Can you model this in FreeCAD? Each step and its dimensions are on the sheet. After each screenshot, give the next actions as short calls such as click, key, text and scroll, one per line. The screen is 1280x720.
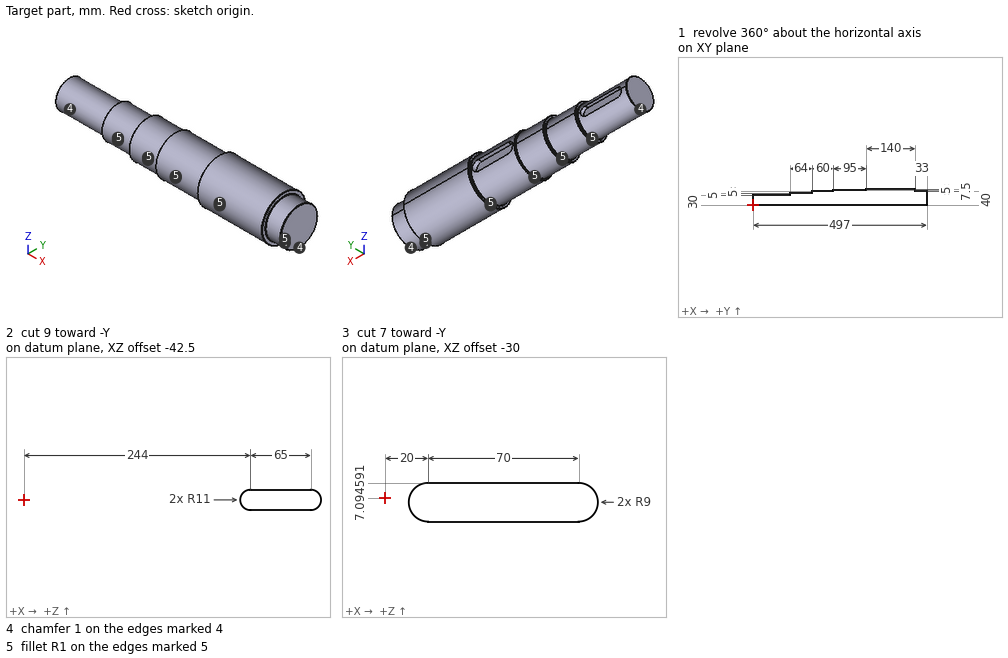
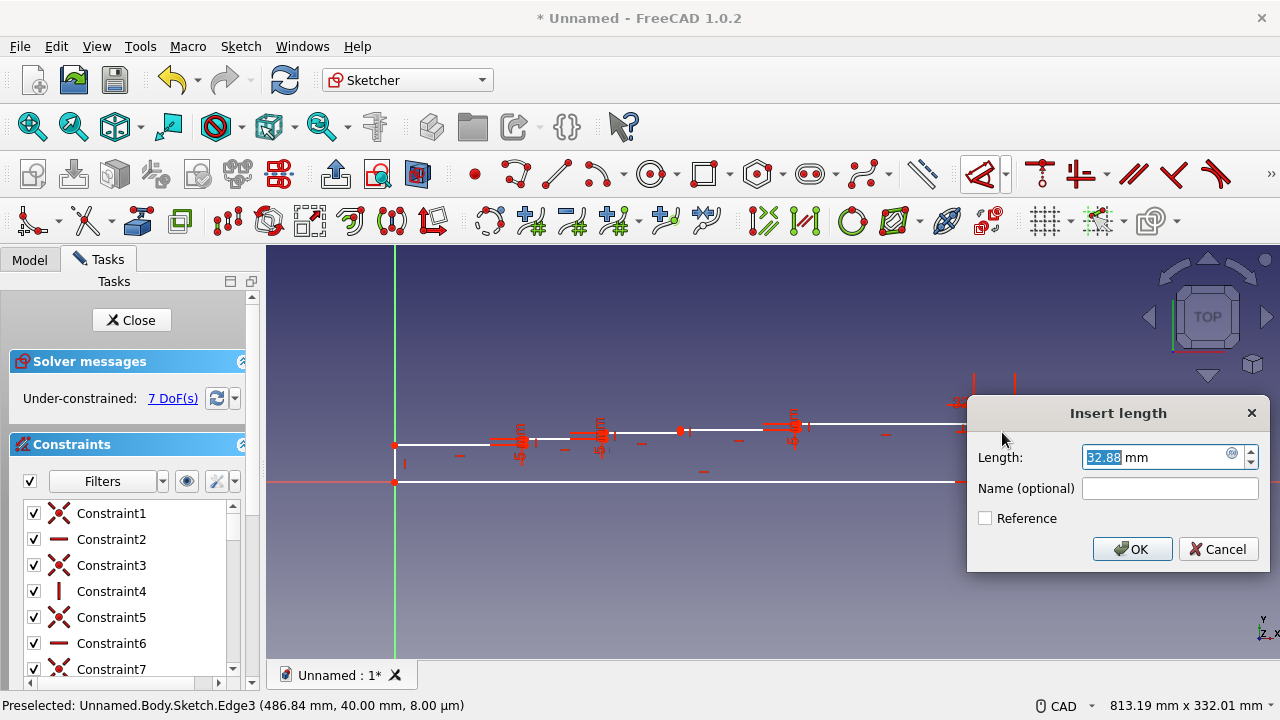
text(33)
key(Return)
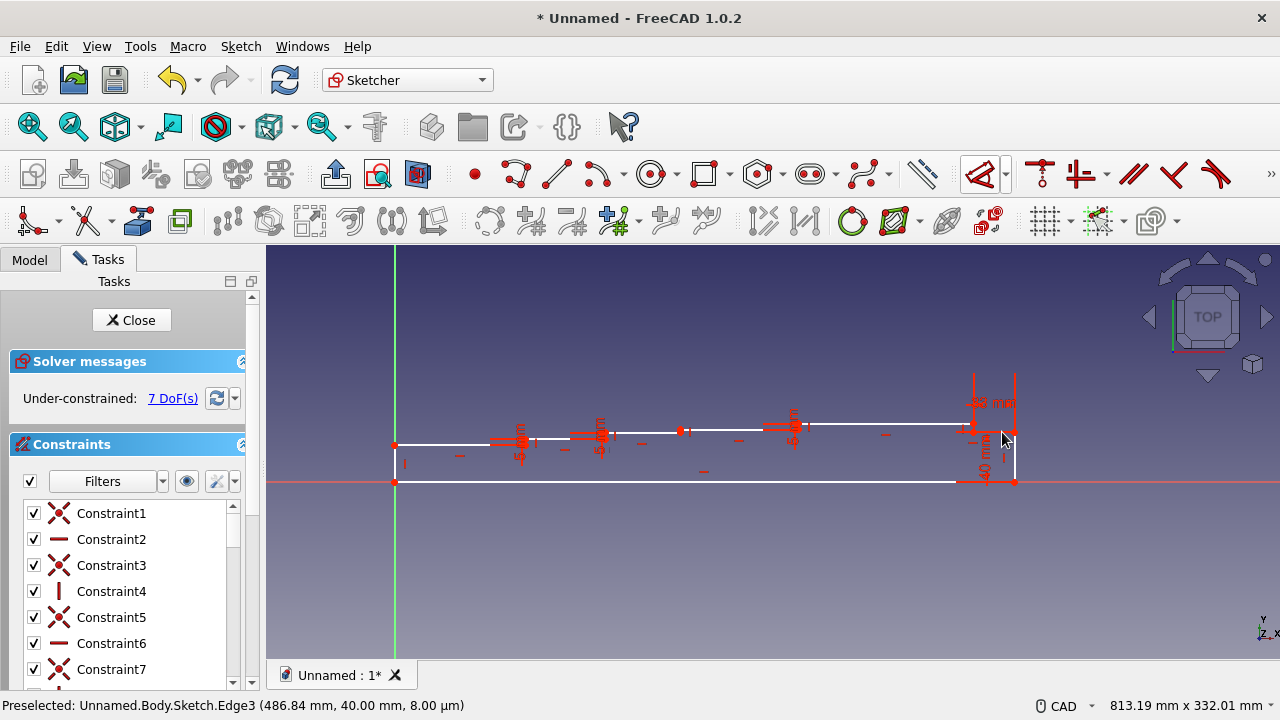
click(763, 430)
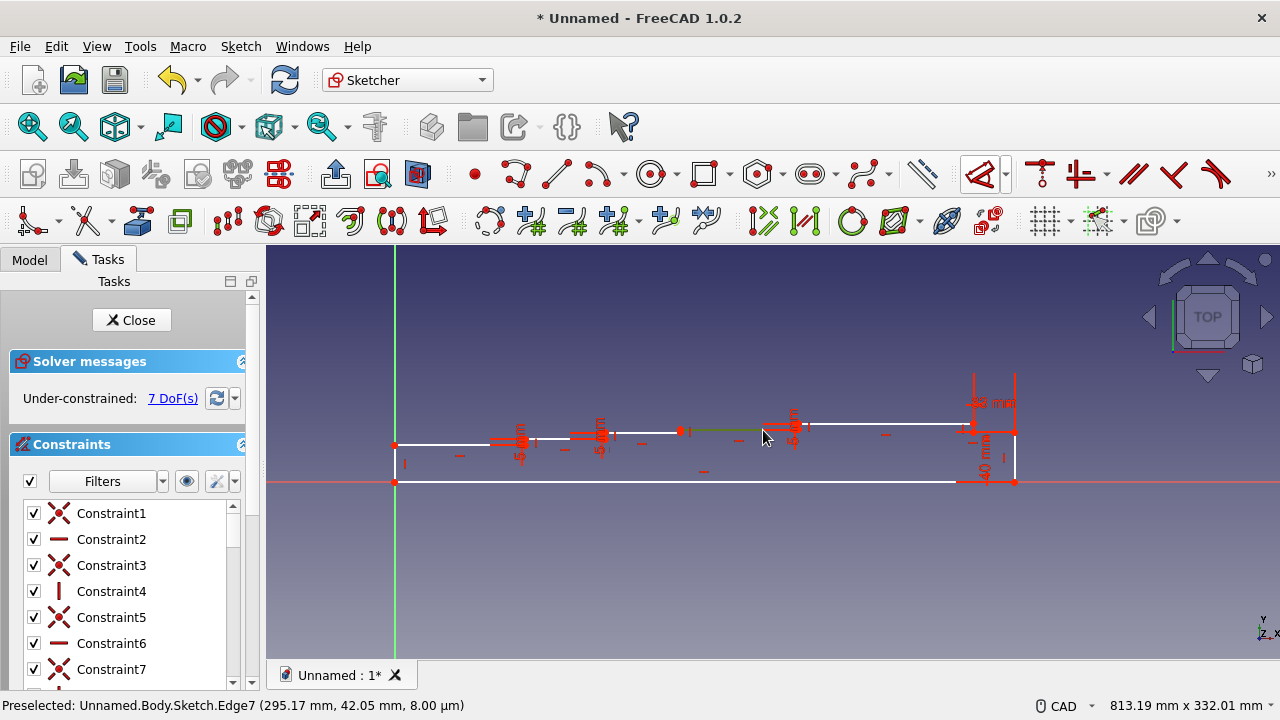
click(1006, 174)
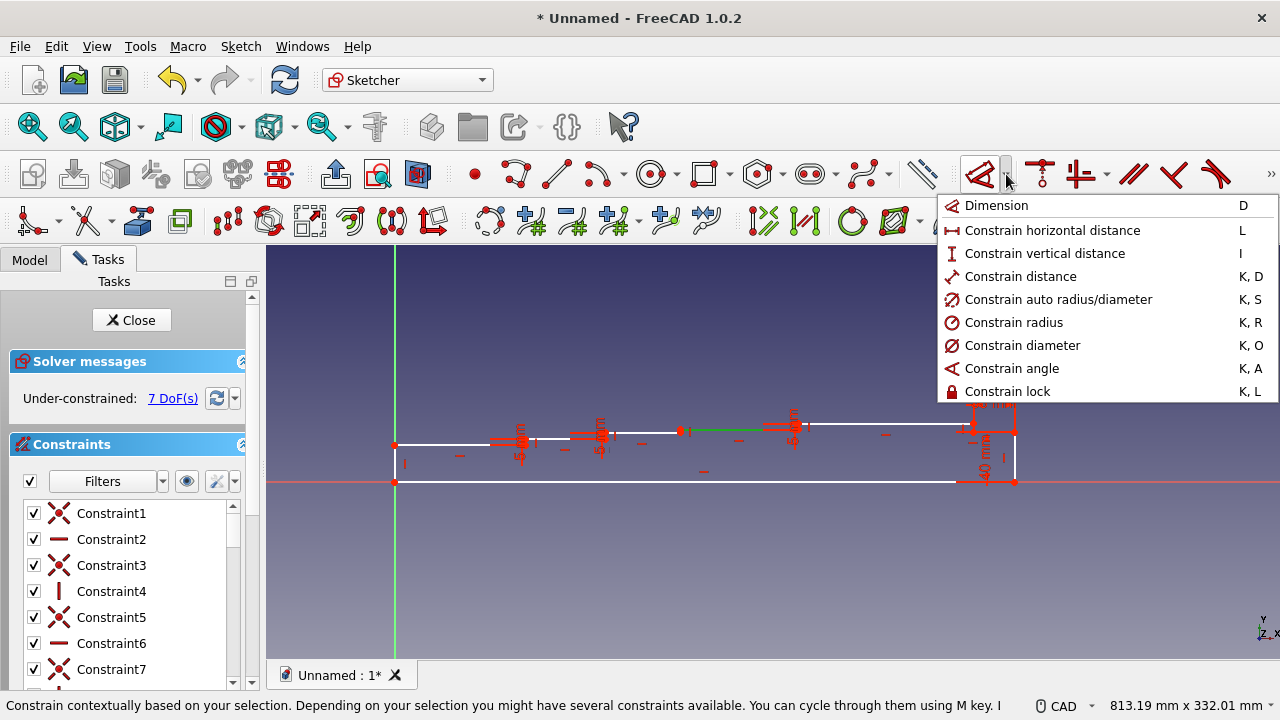
click(1108, 230)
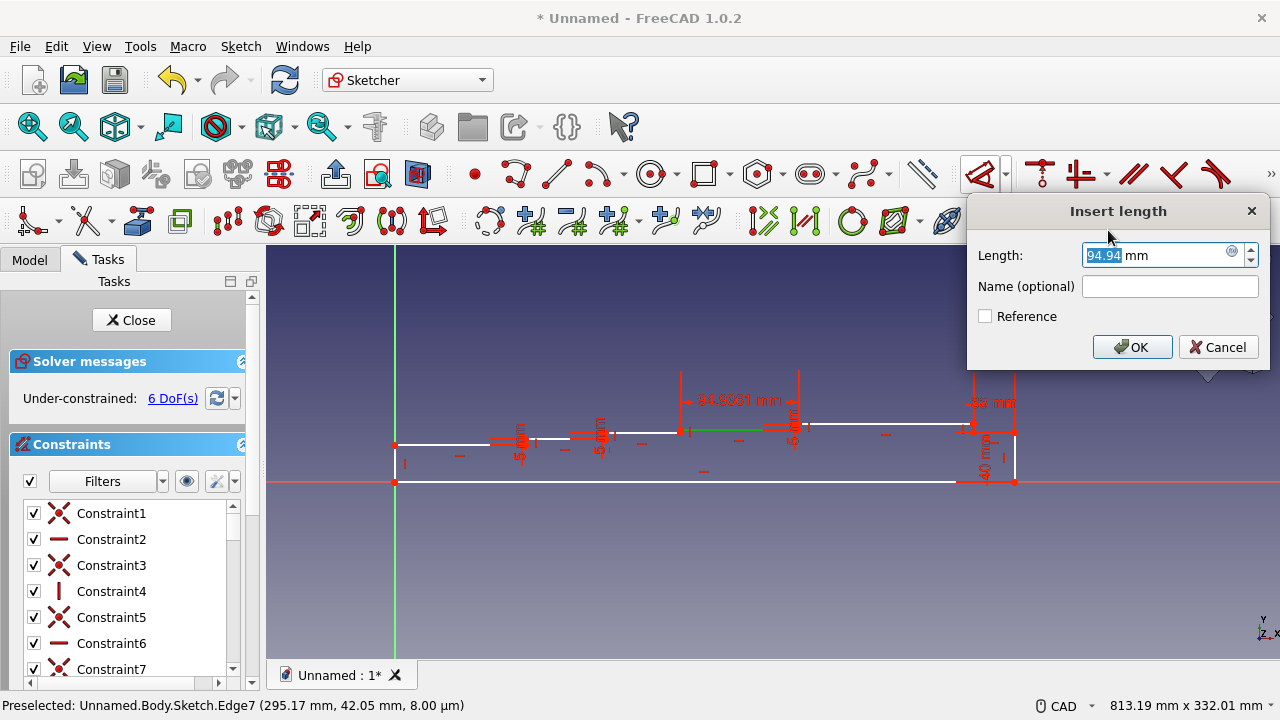
text(95)
key(Return)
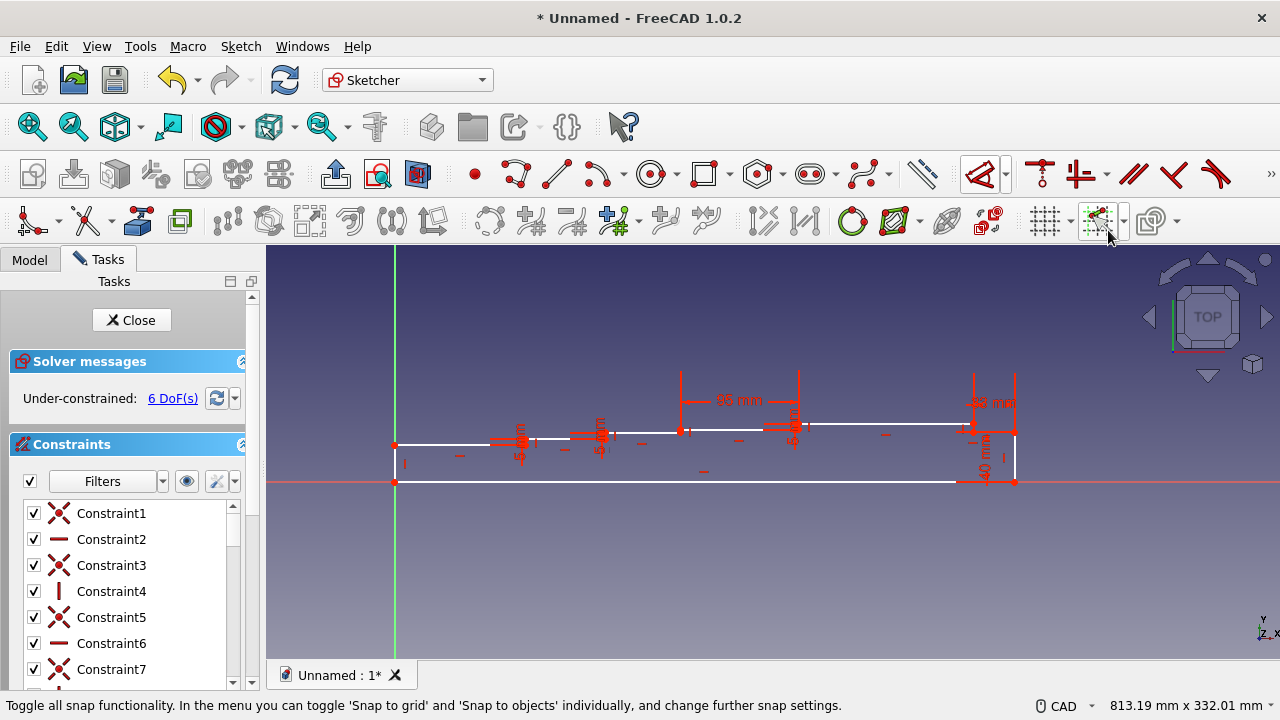
click(658, 433)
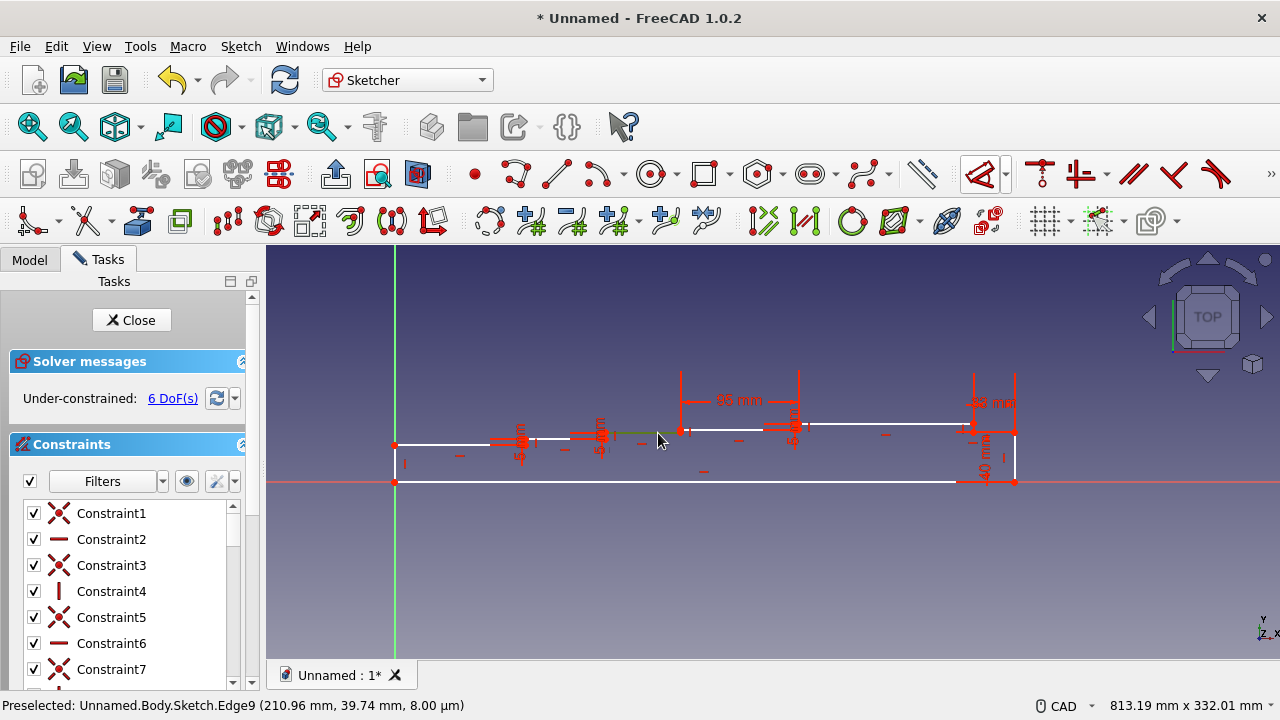
key(l)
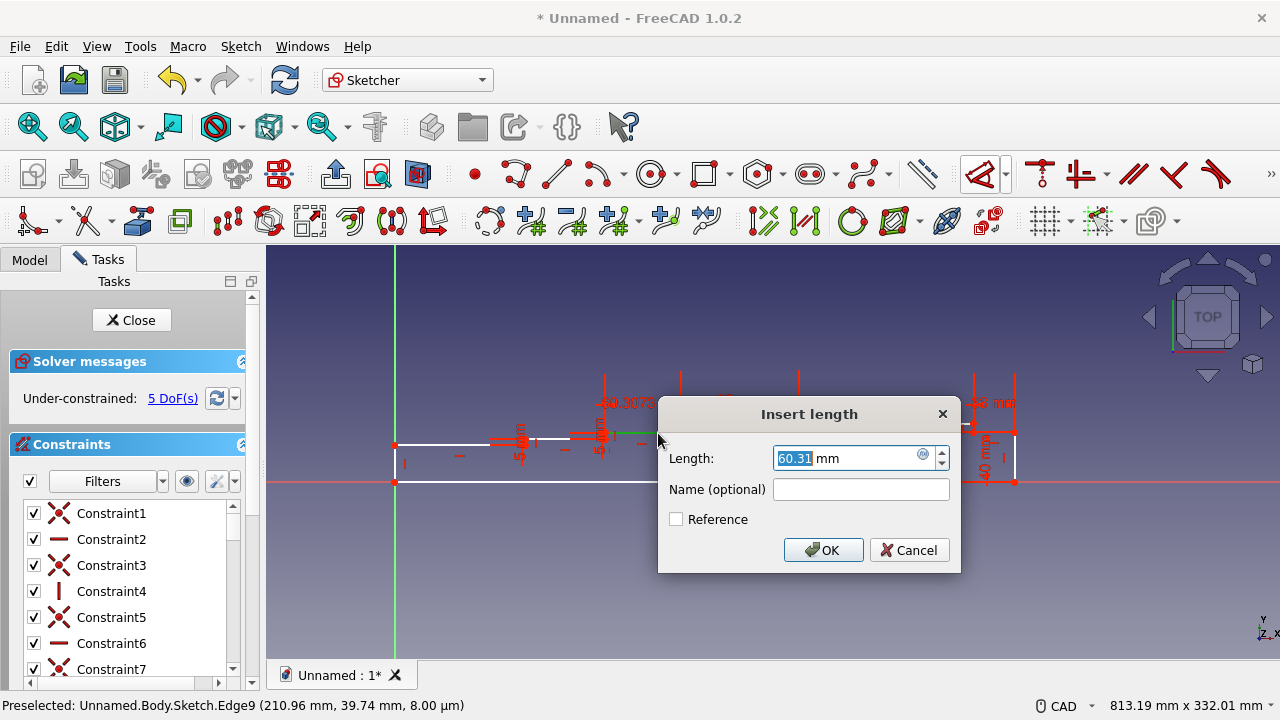
text(60)
key(Return)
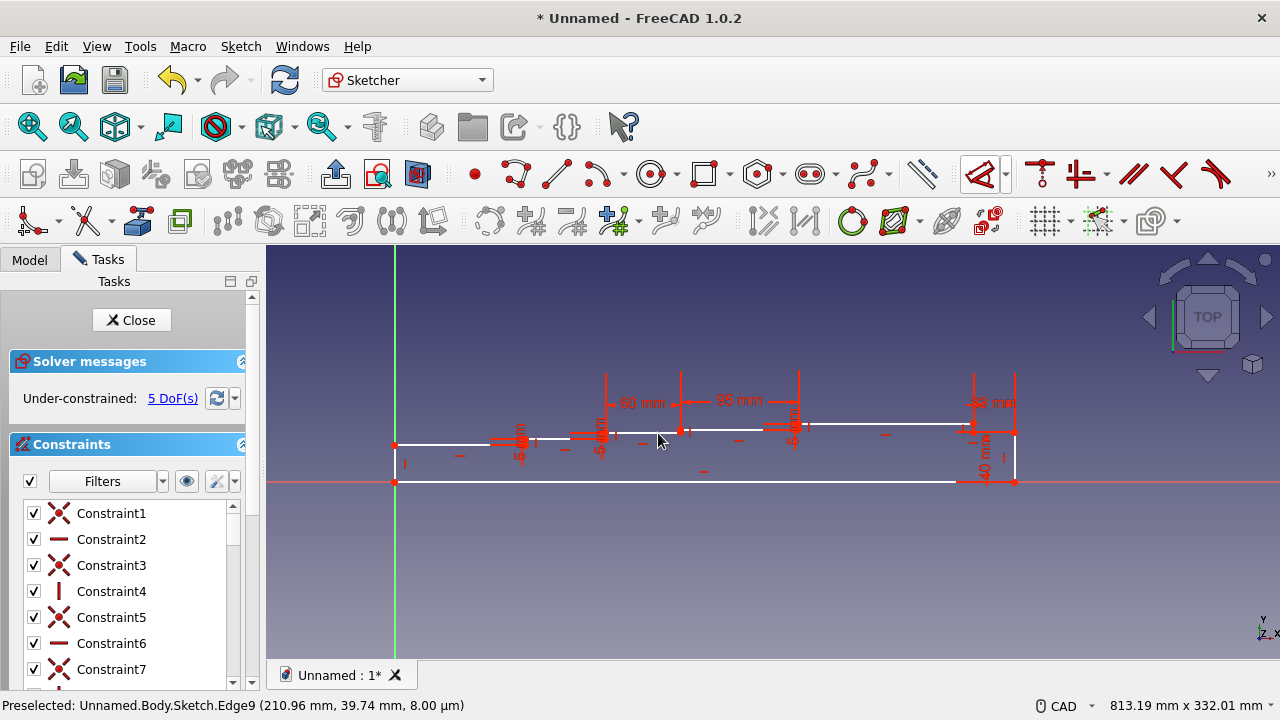
click(582, 439)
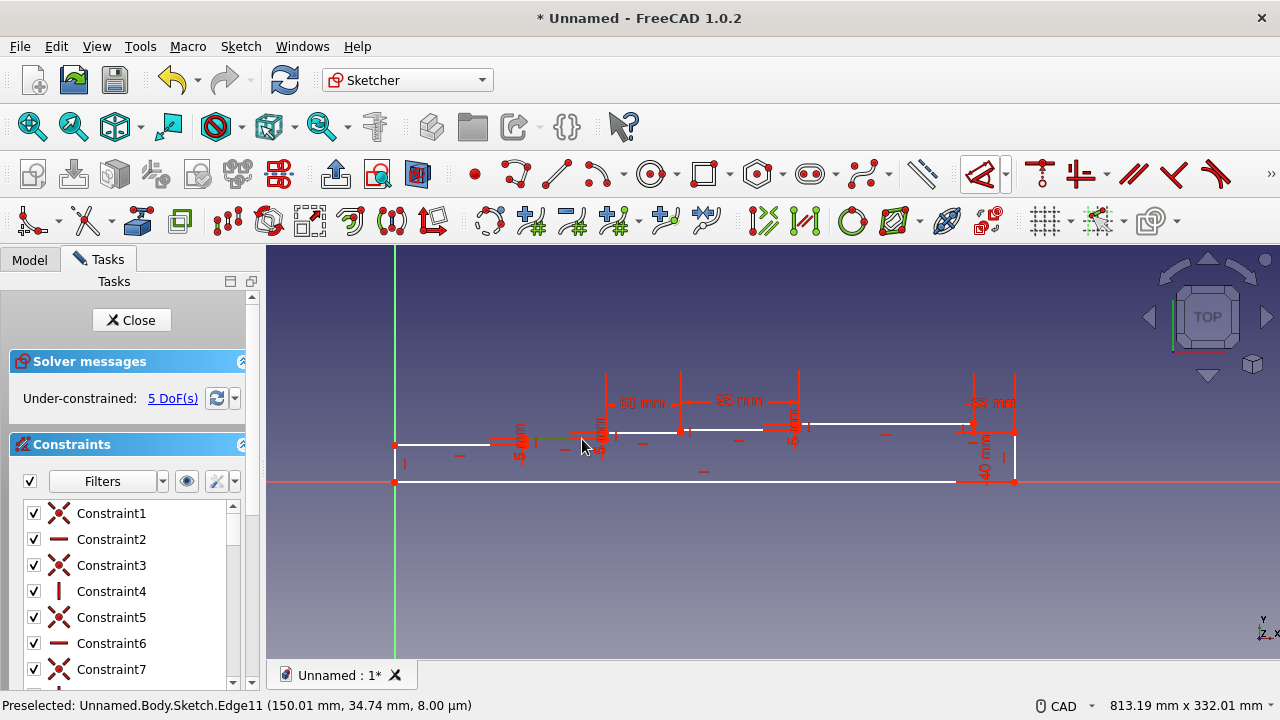
click(1006, 174)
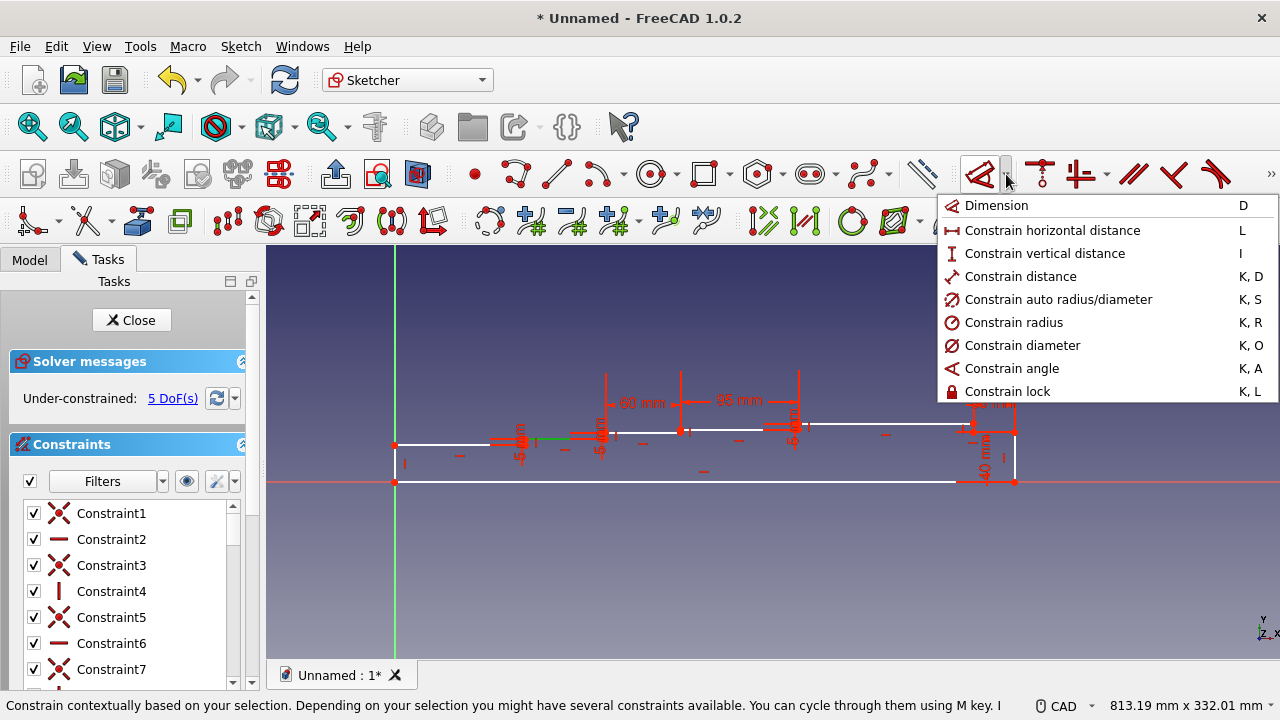
click(1108, 230)